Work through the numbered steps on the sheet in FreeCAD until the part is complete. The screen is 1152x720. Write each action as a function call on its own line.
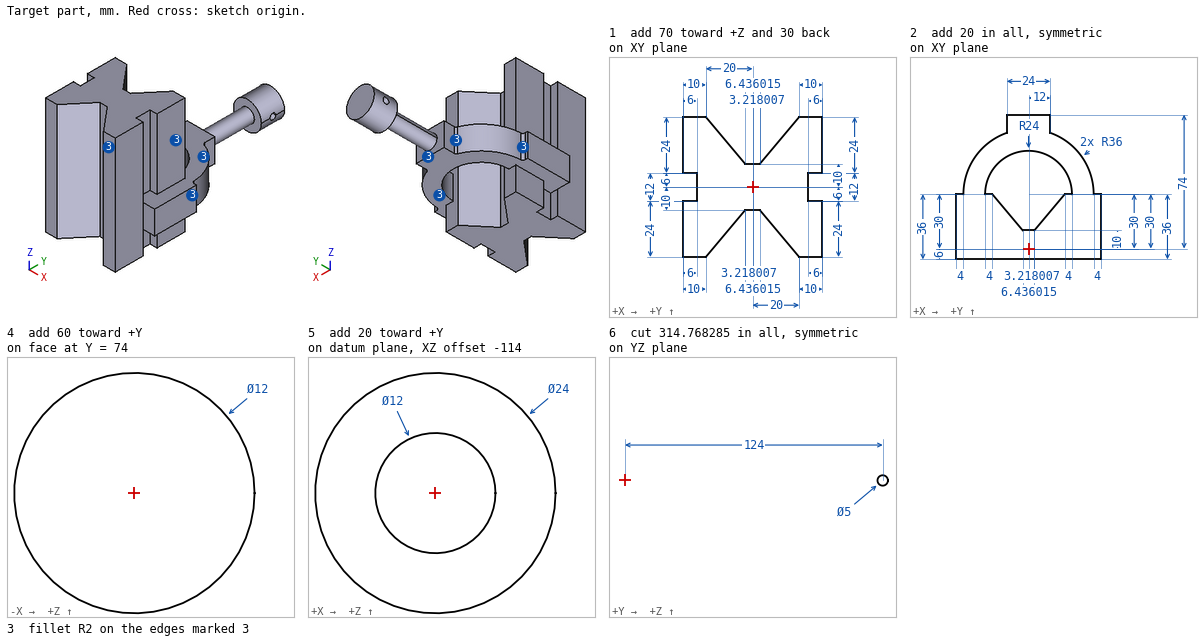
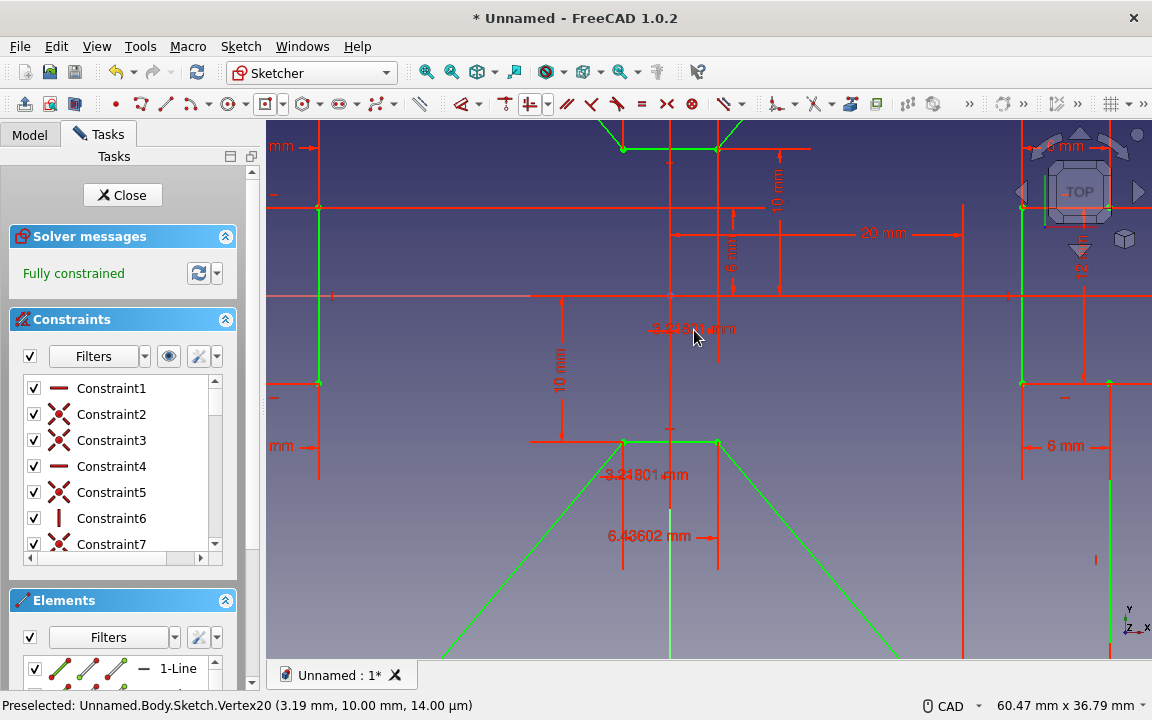
click(123, 195)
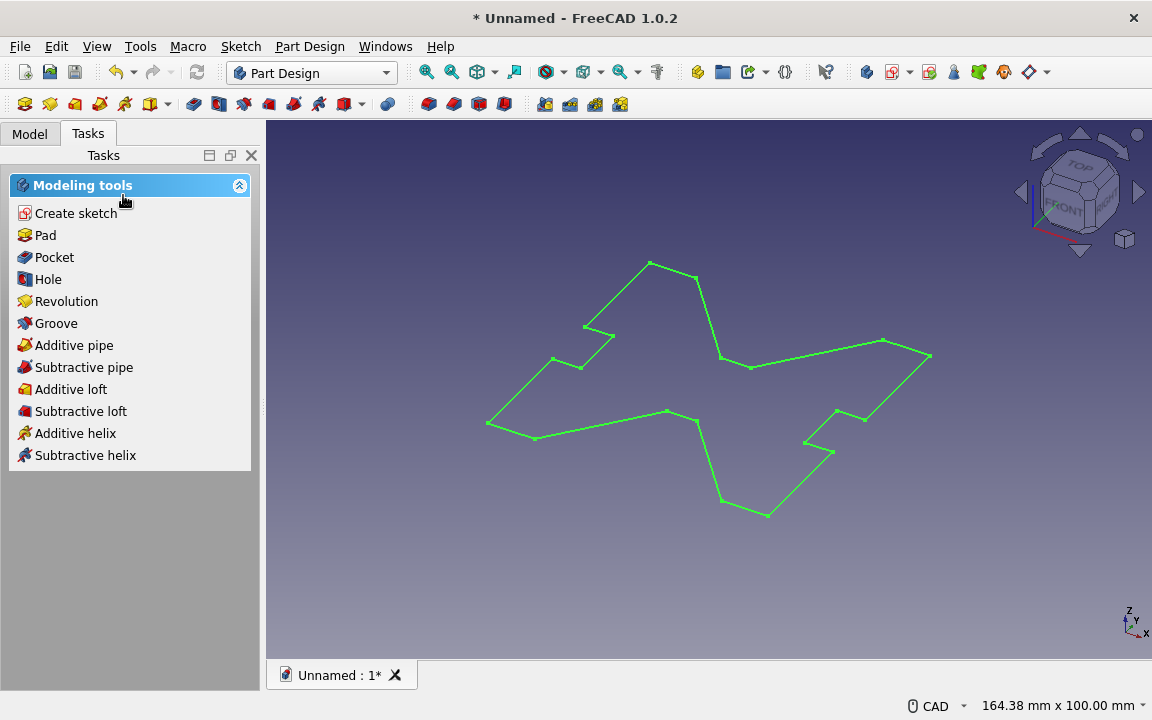
click(25, 104)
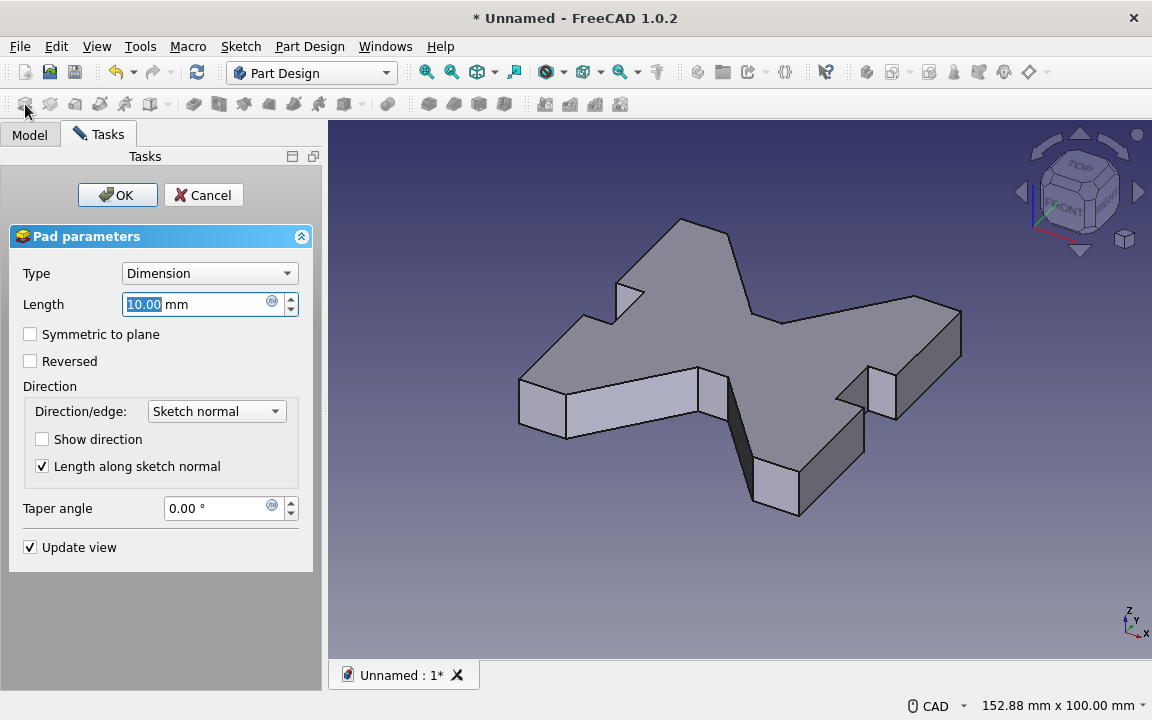
click(210, 274)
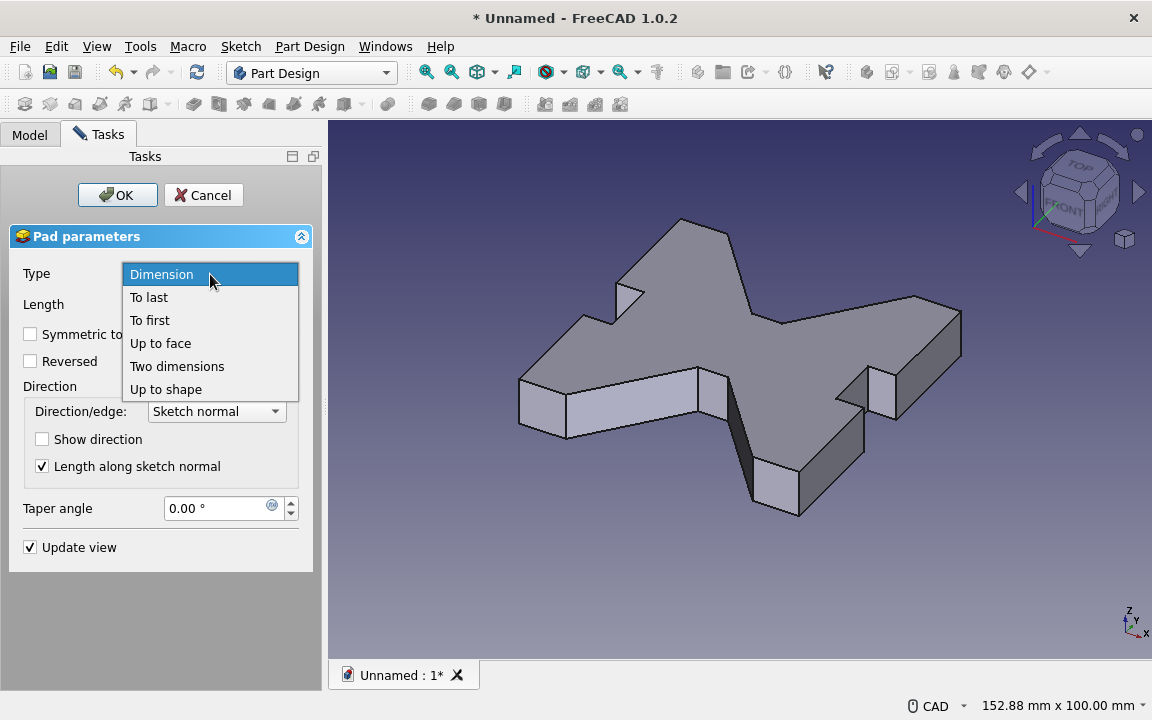
click(208, 366)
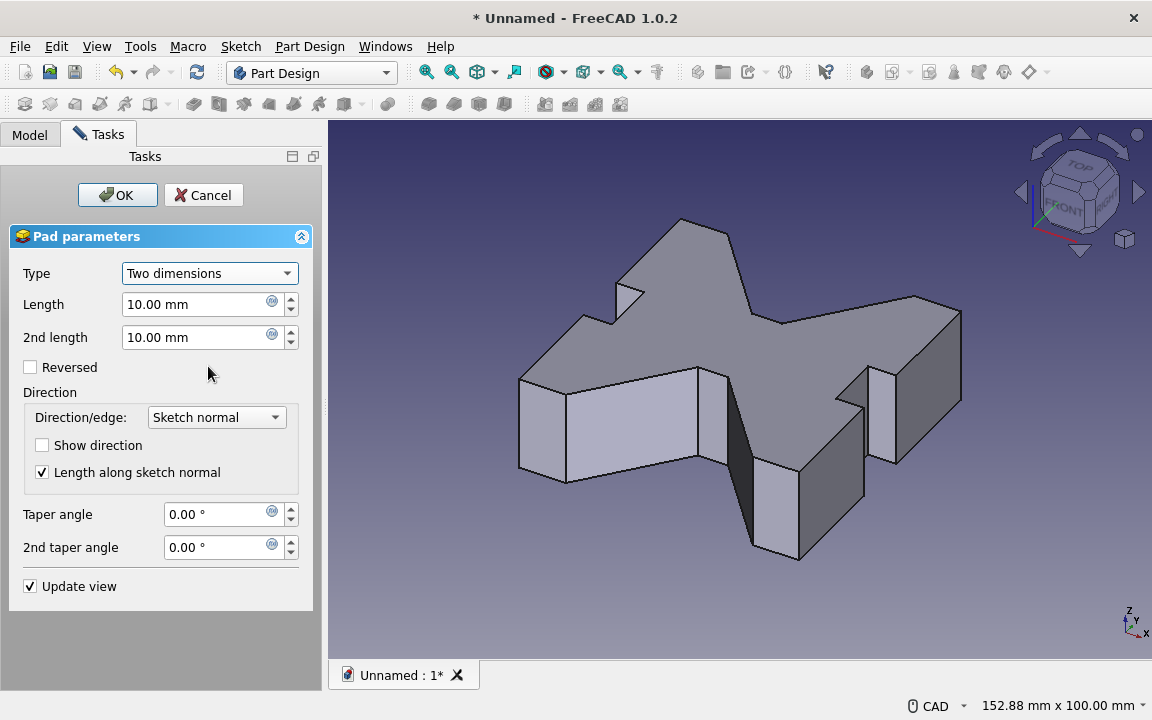
triple_click(204, 304)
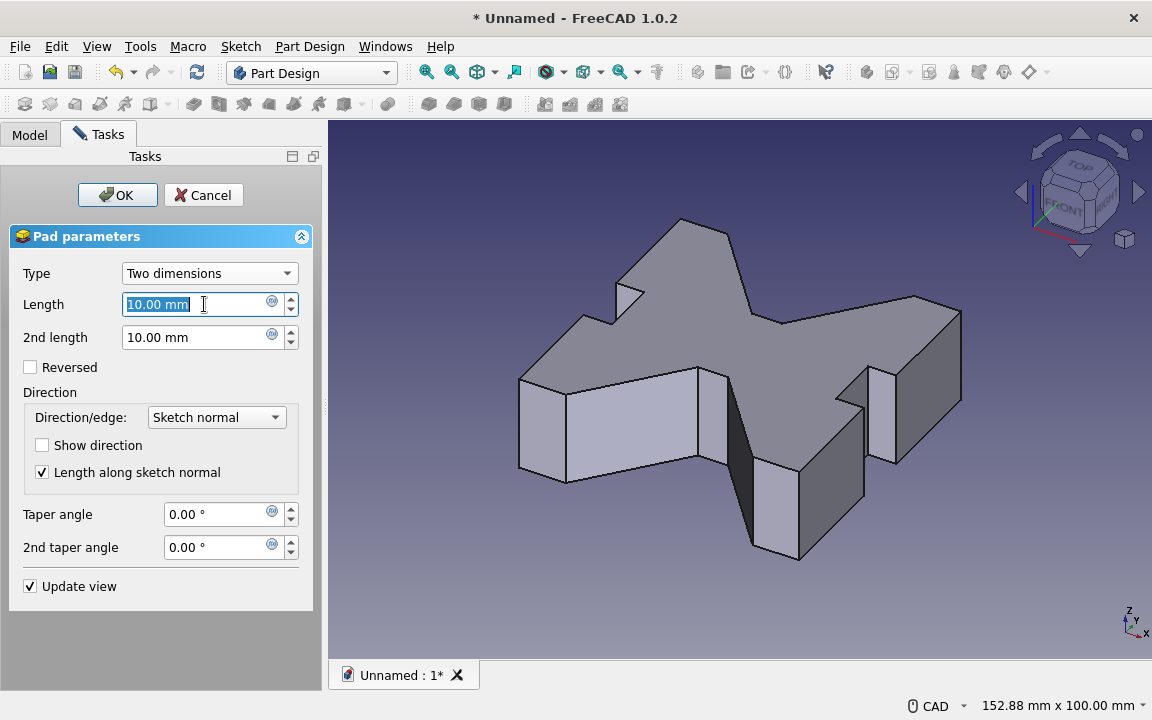
text(70)
key(Tab)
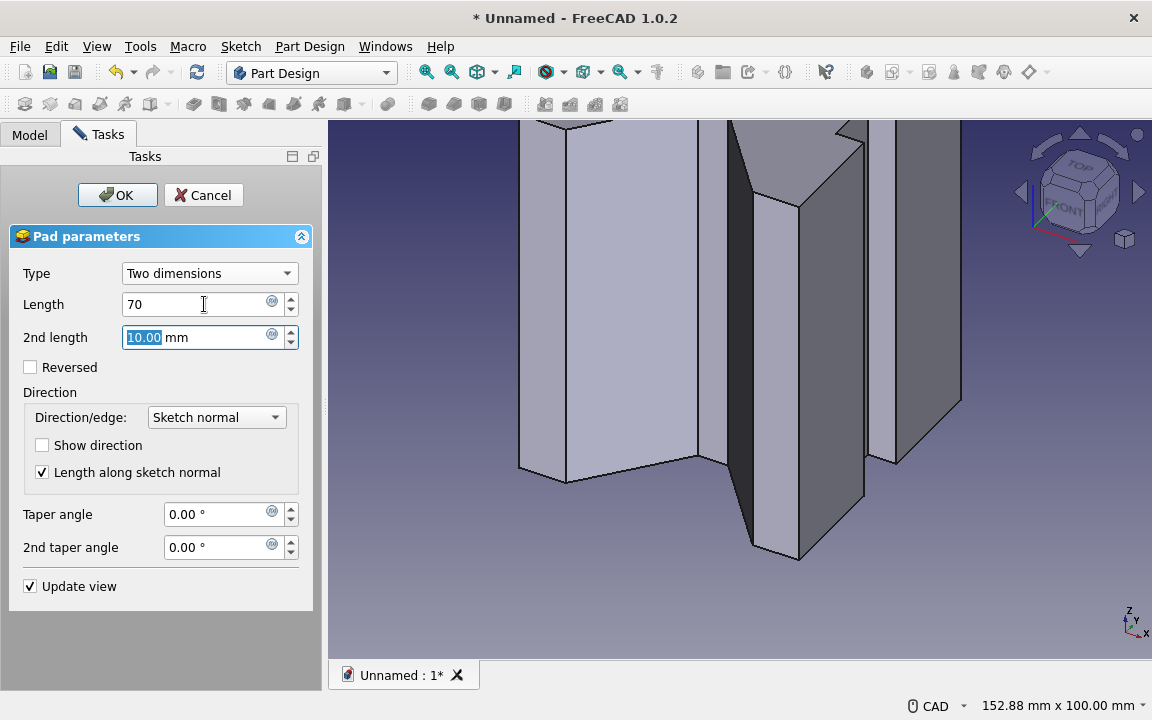
text(30)
key(Tab)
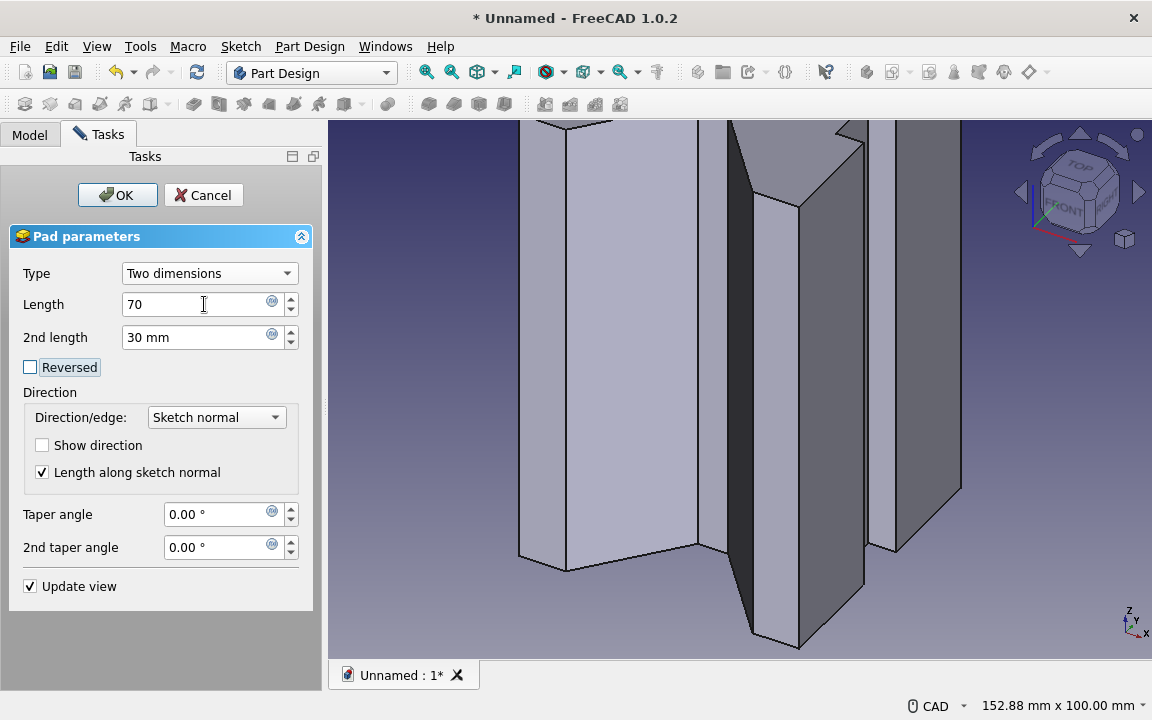
click(118, 195)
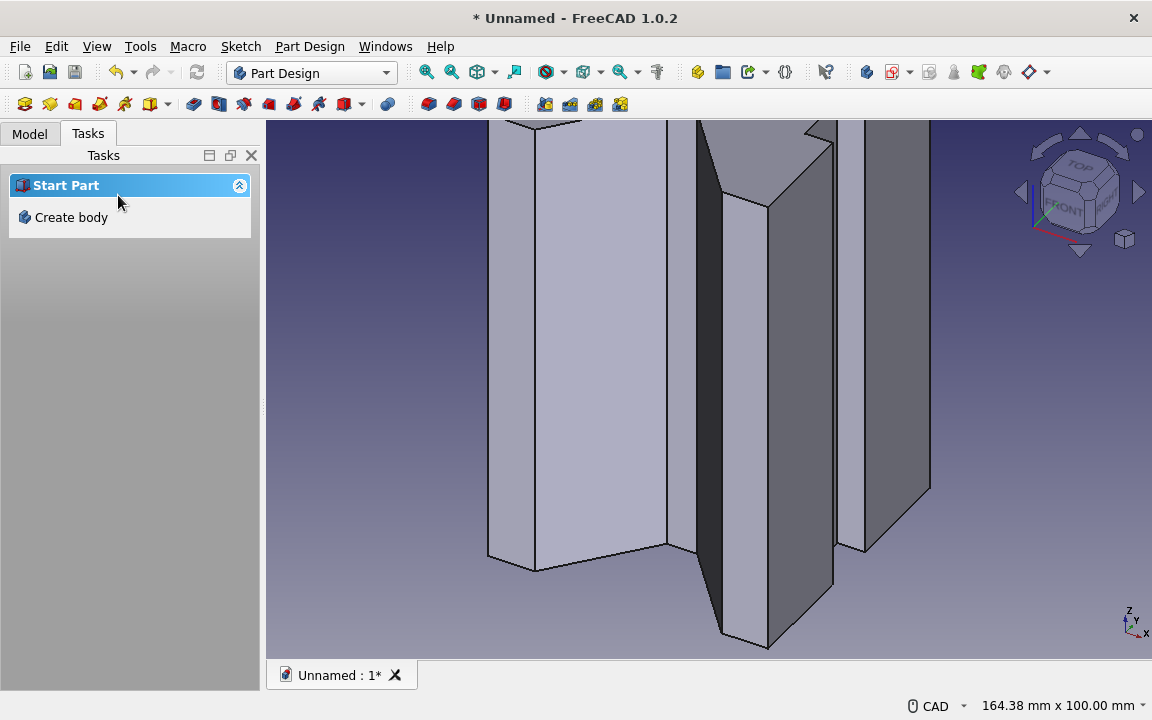
click(427, 72)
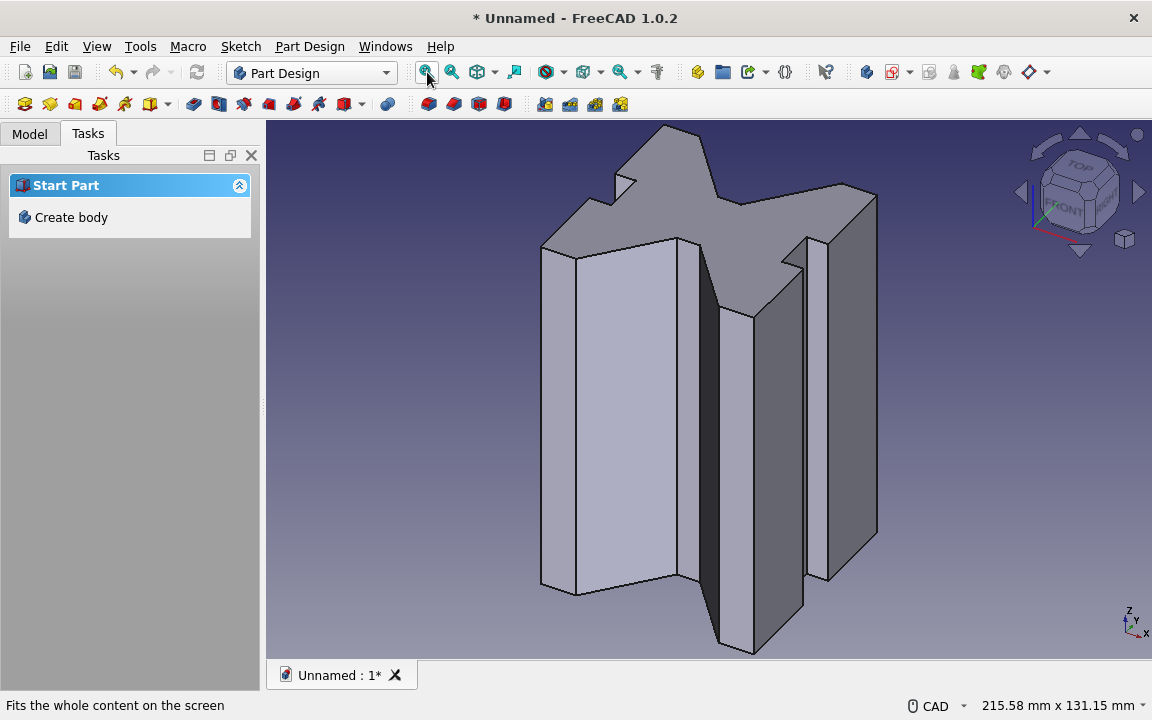
click(892, 72)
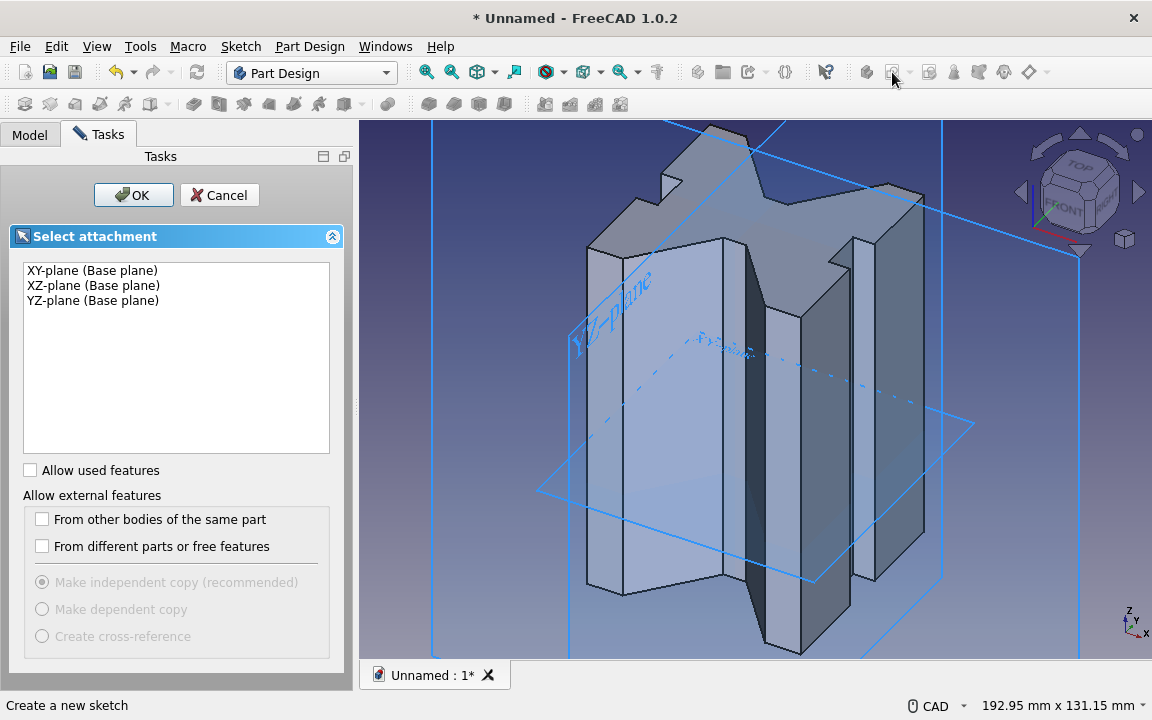
click(84, 270)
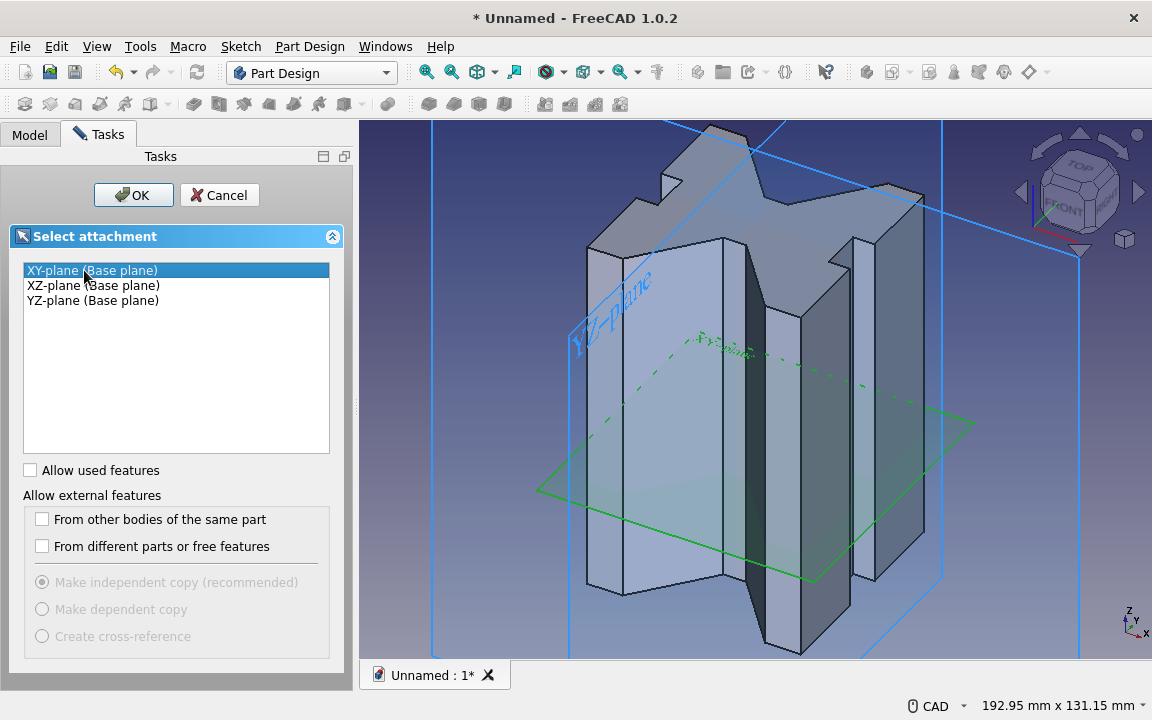
click(134, 195)